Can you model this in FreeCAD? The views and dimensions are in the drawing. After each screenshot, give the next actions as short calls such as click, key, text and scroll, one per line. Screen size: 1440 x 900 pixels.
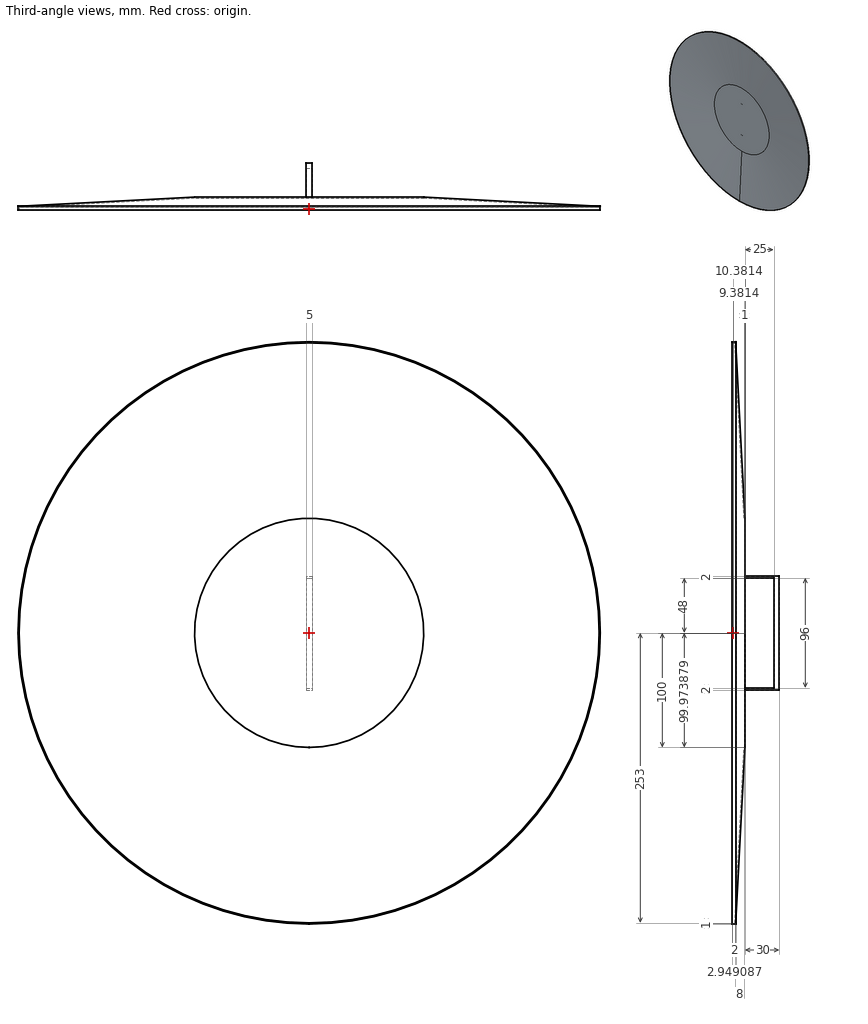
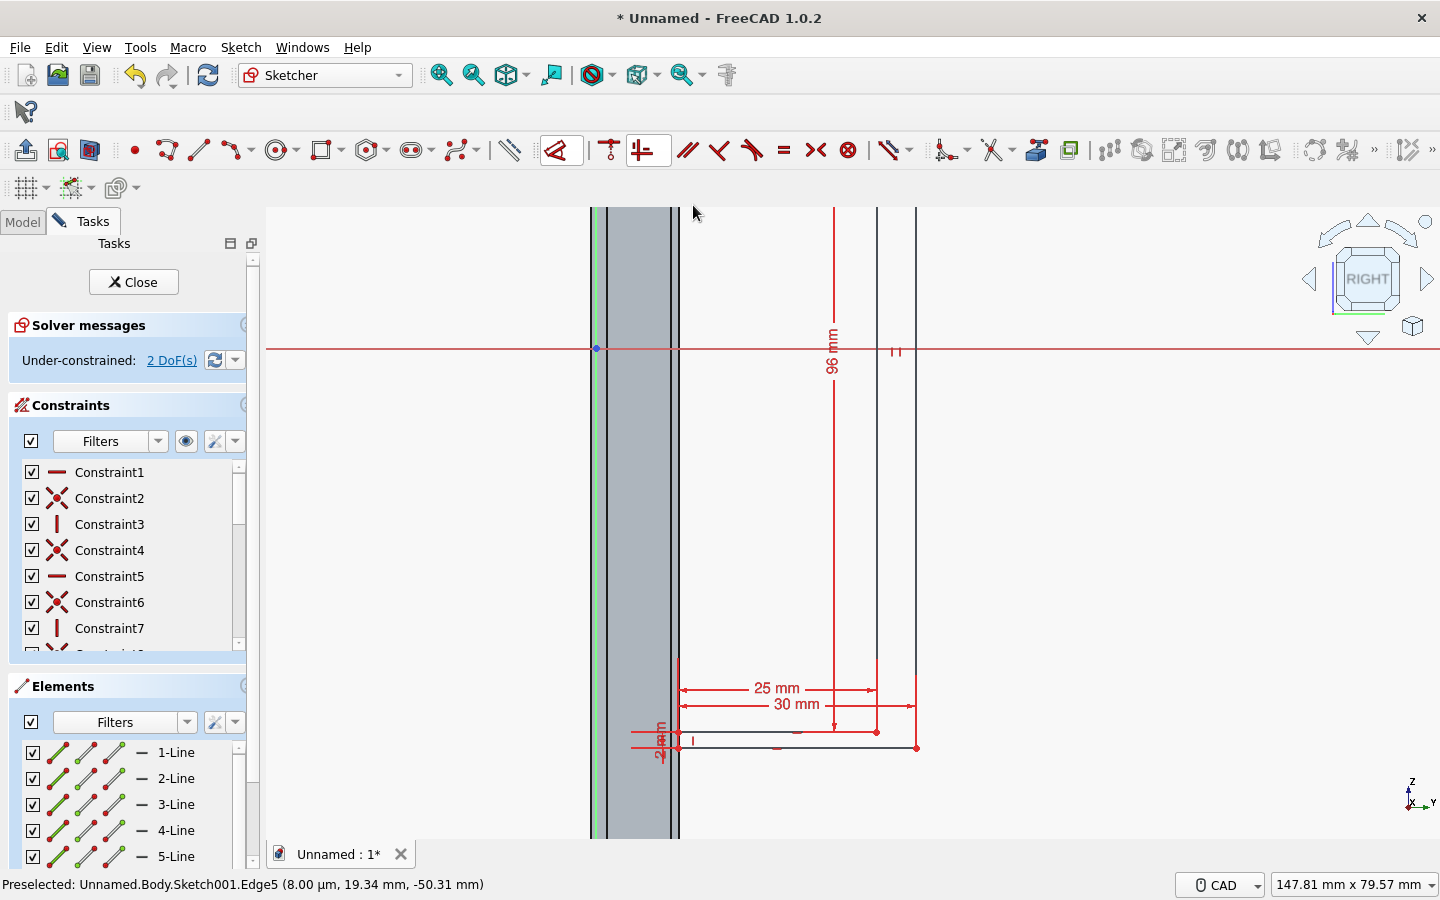
scroll(818, 735, down, 3)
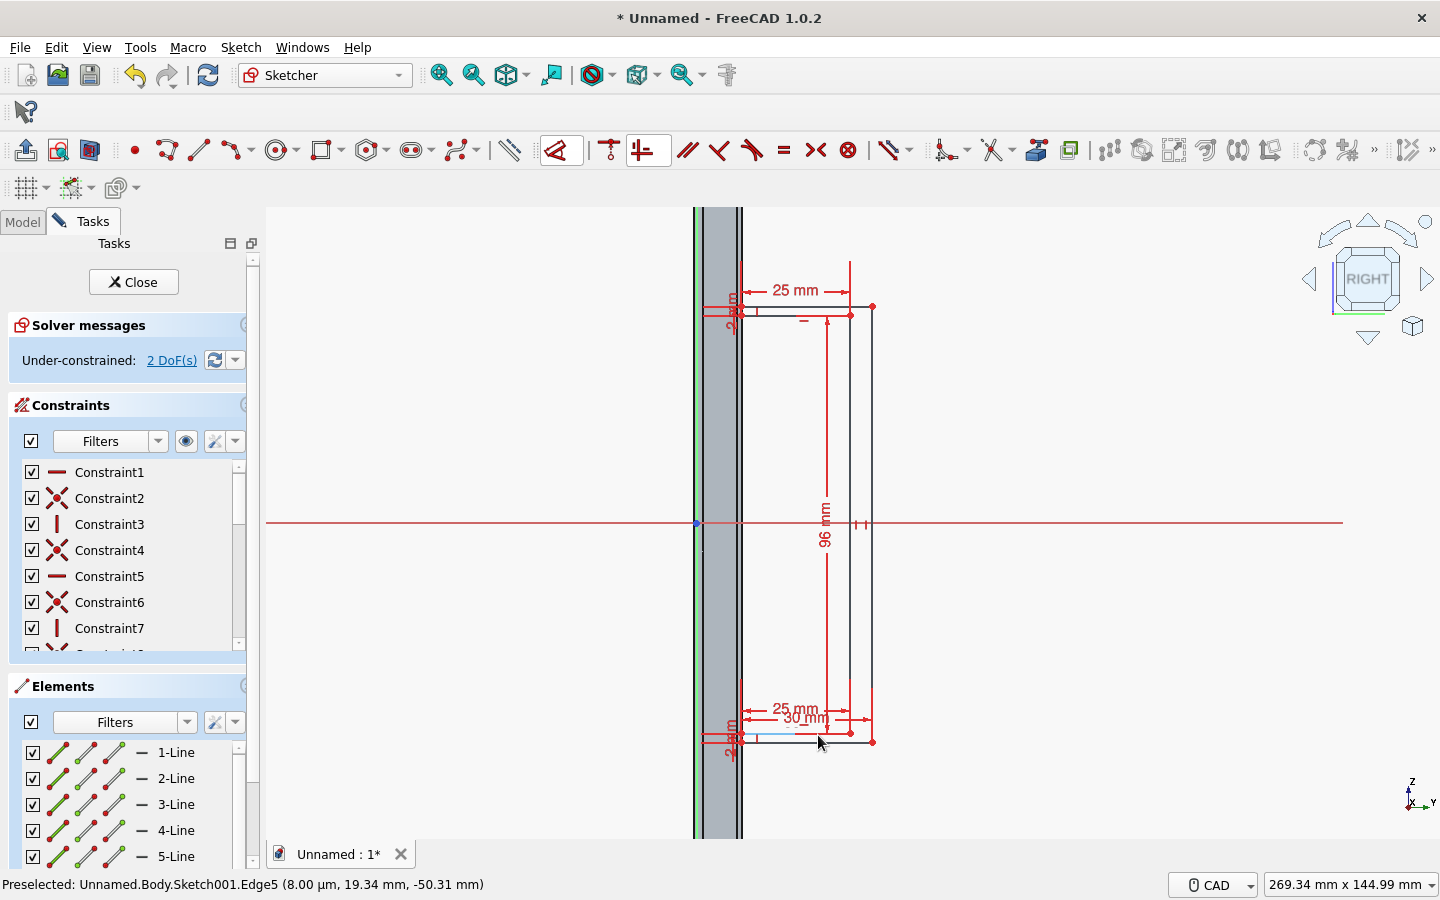
scroll(741, 316, up, 2)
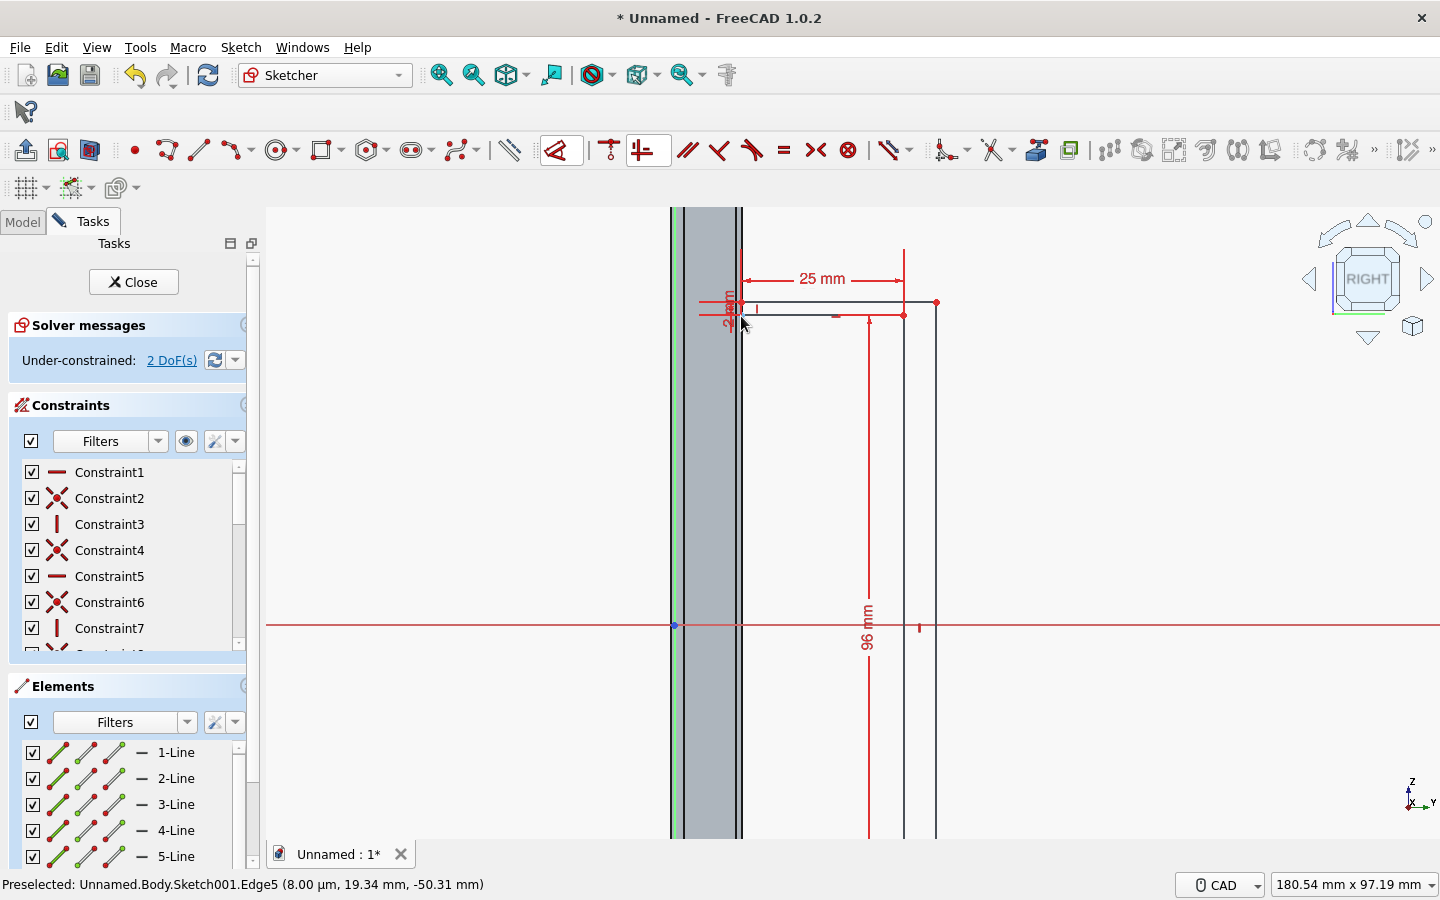
click(741, 315)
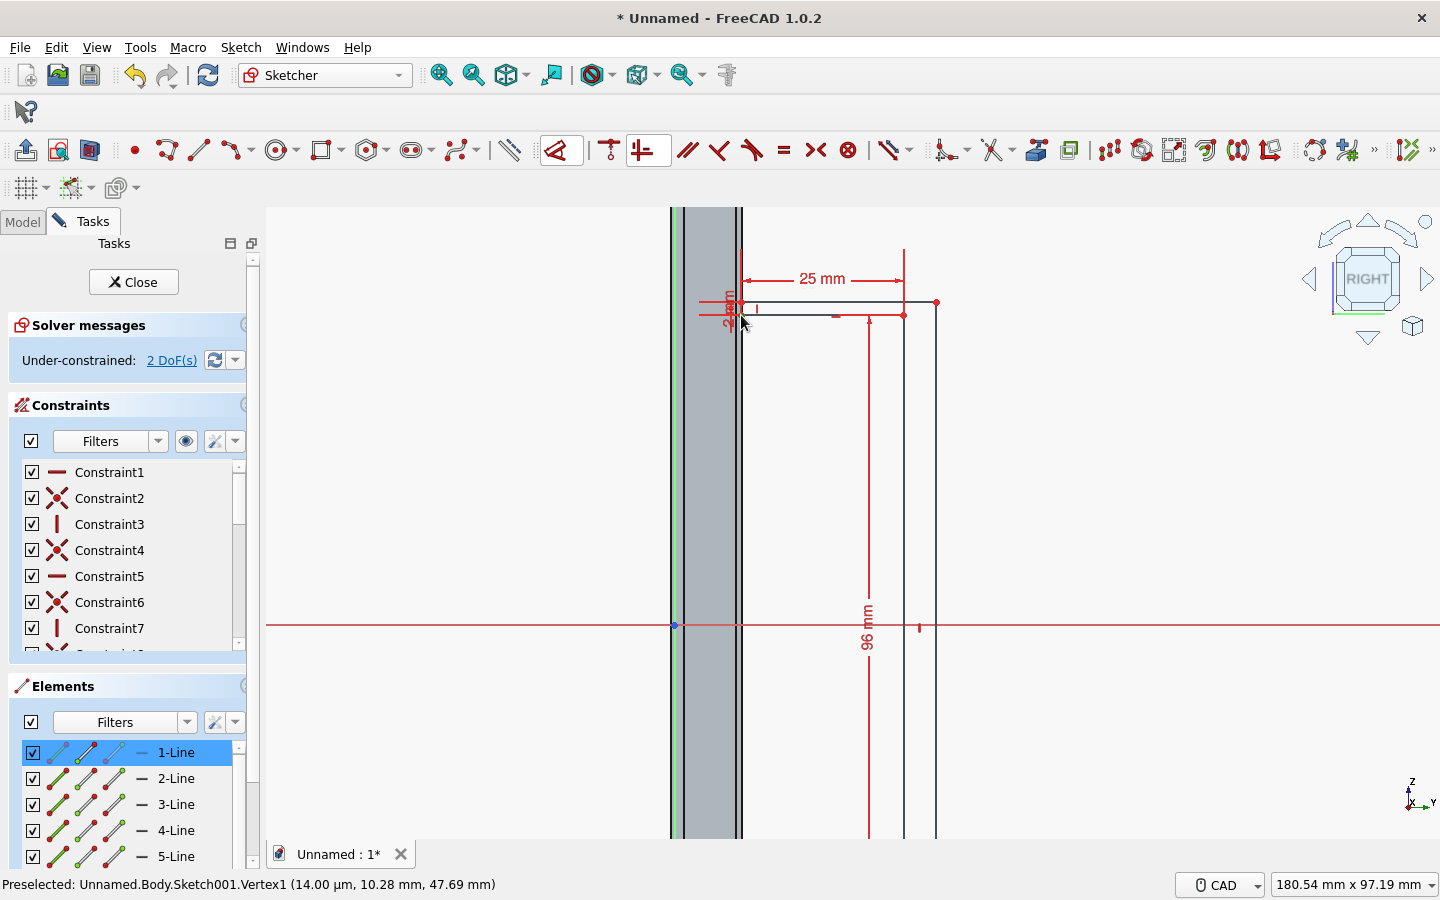
key(i)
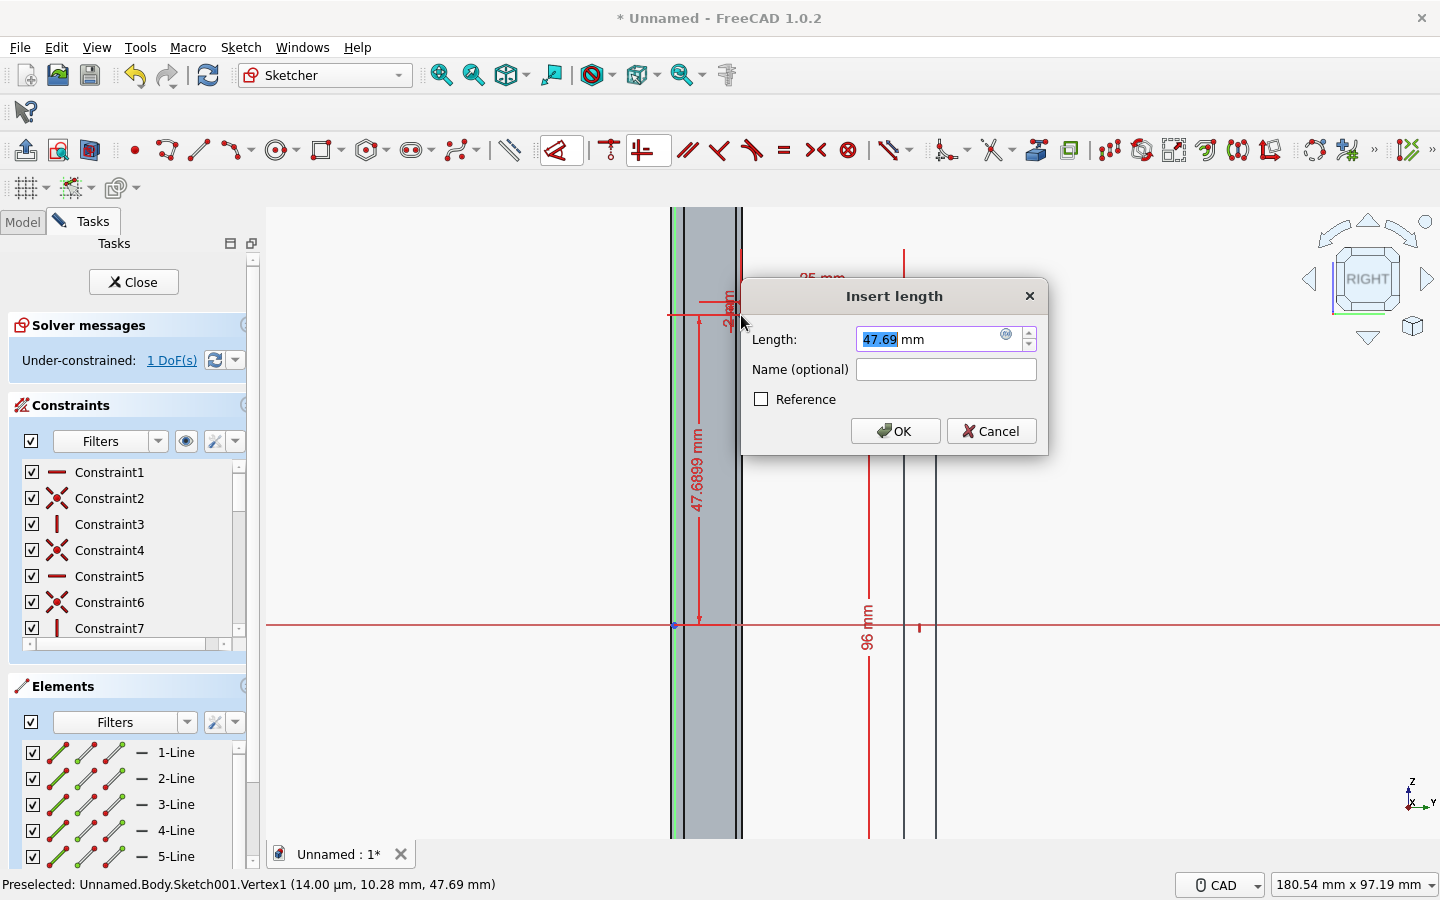
text(48)
key(Return)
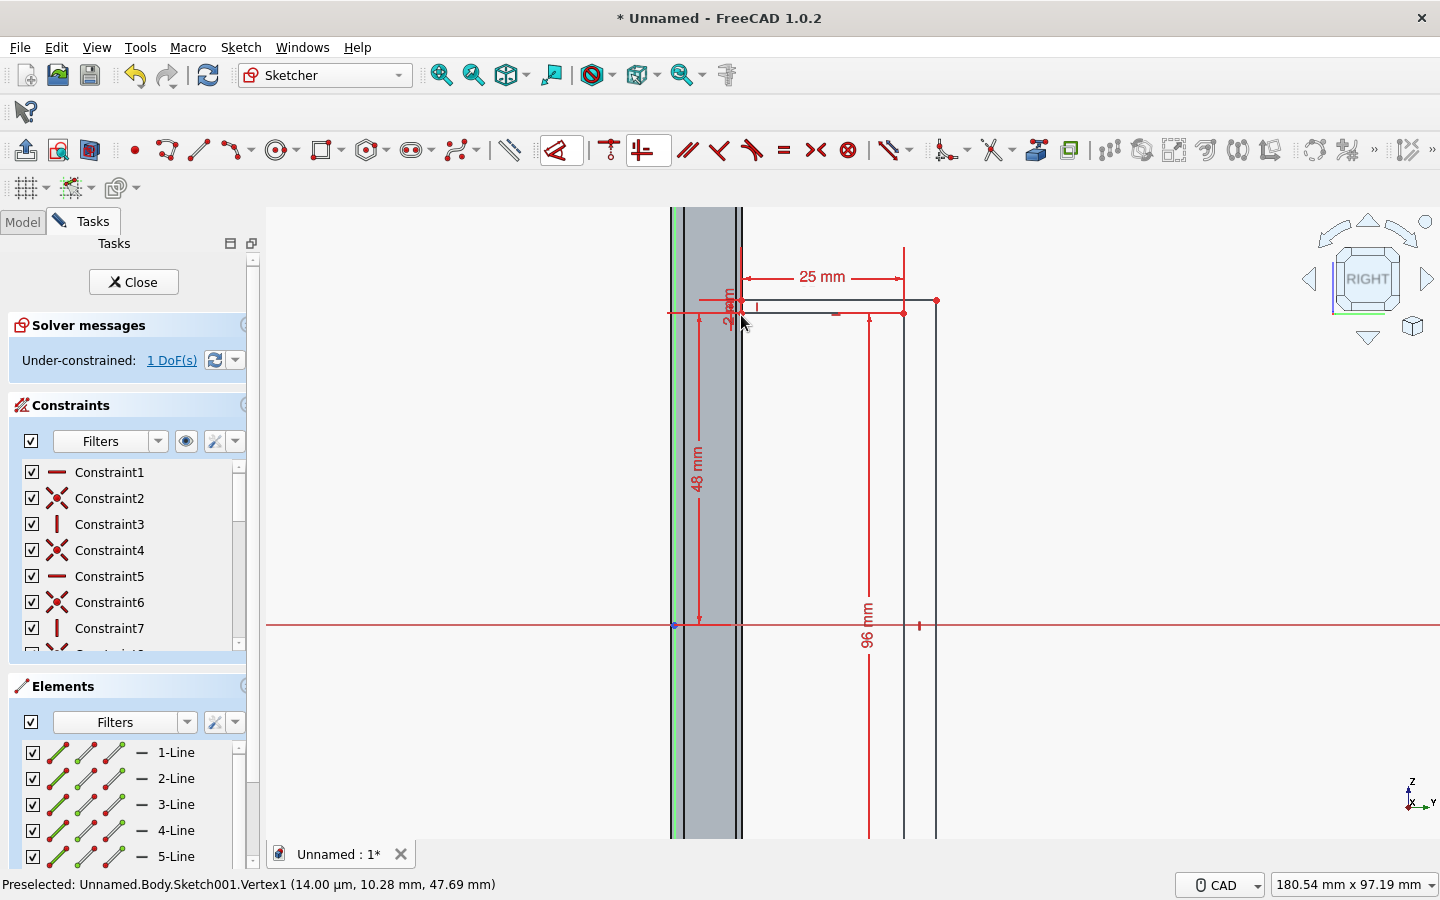
click(741, 313)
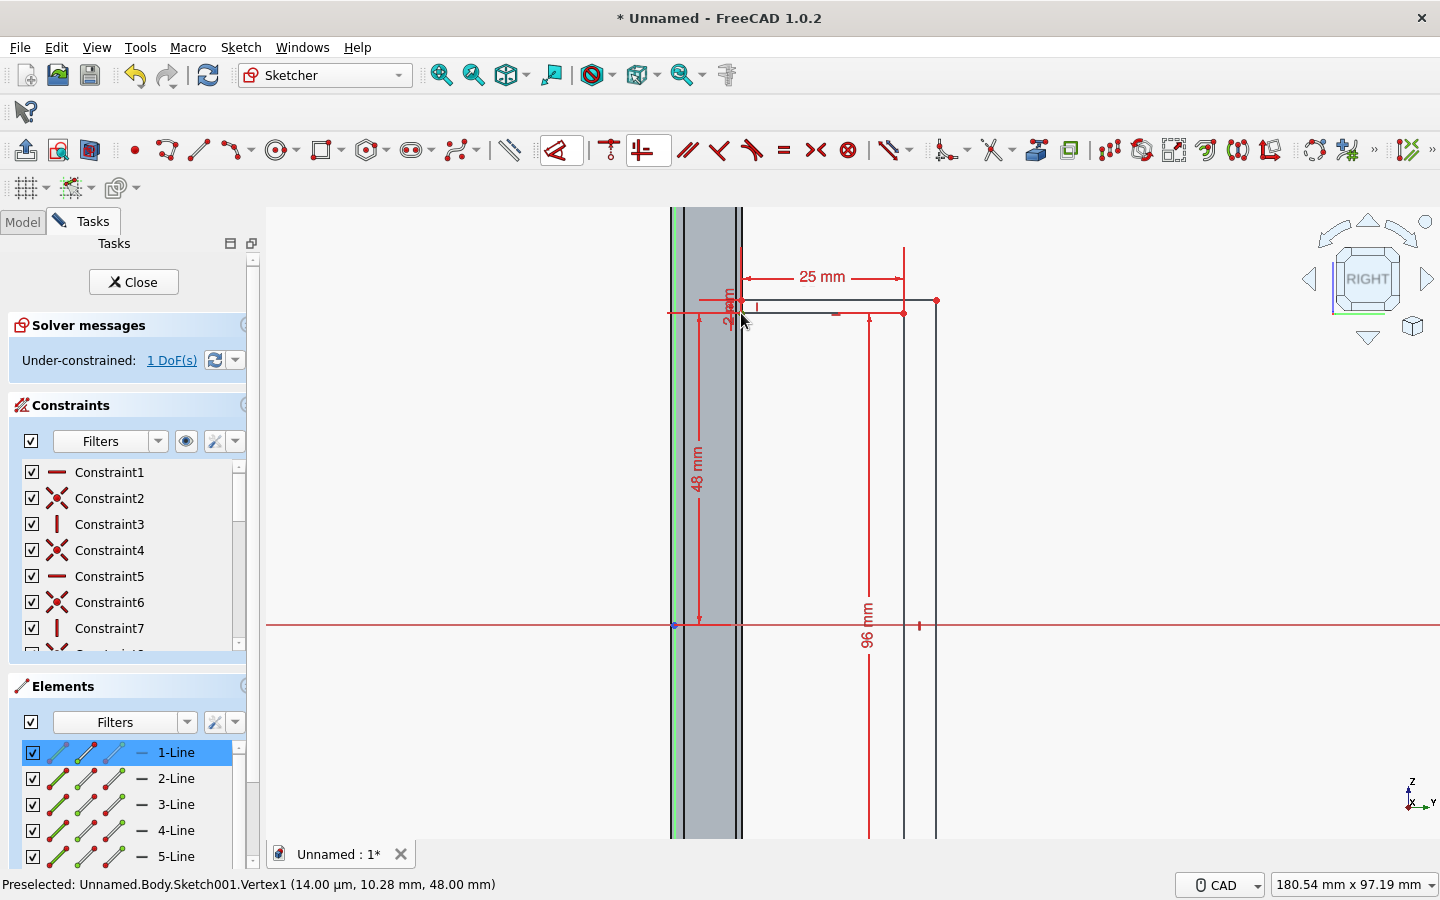
click(578, 150)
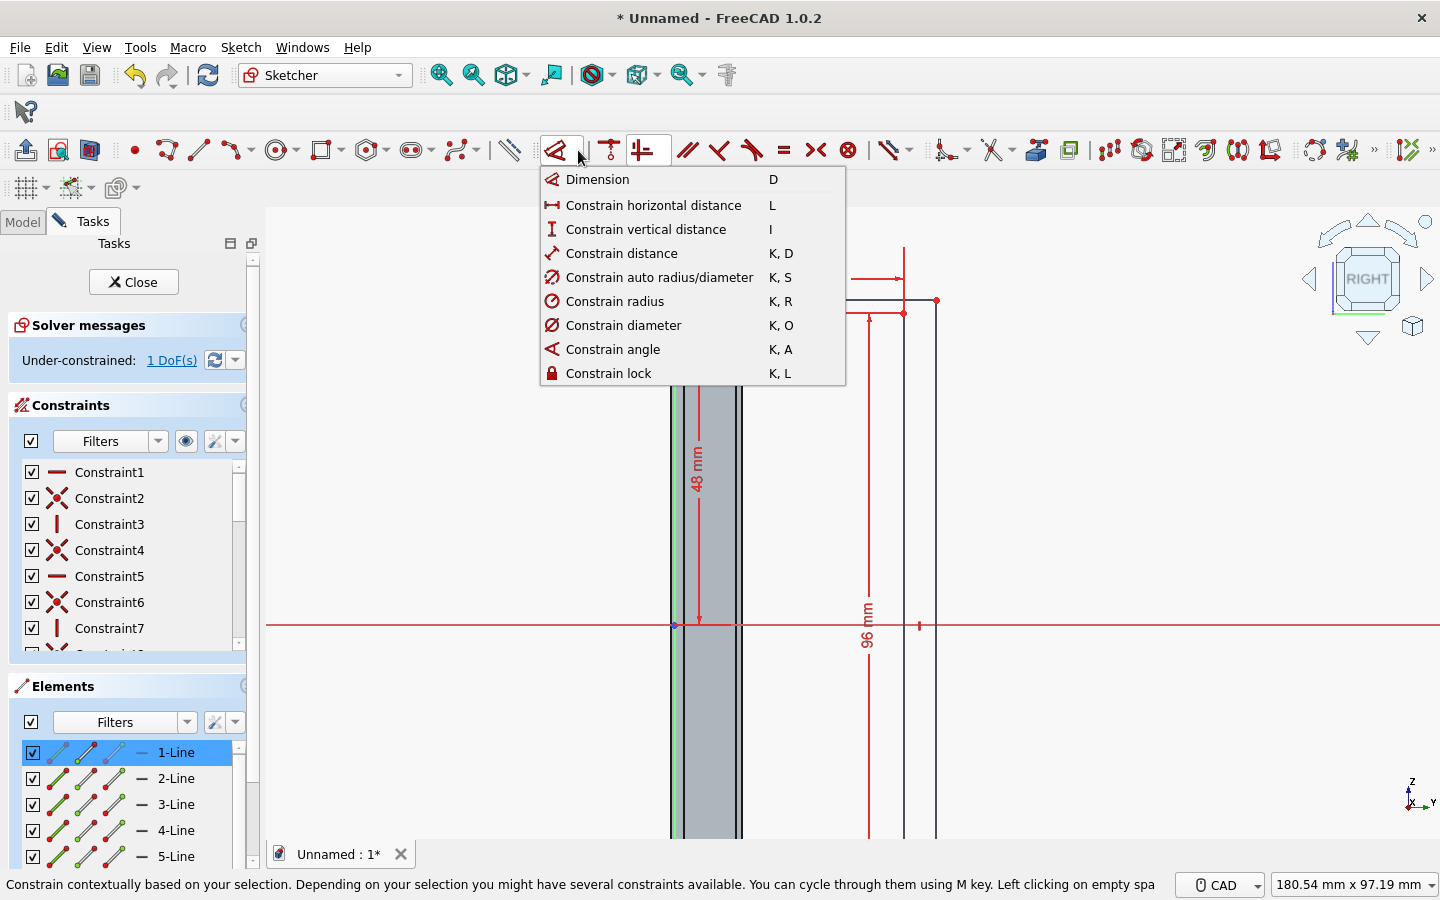
click(693, 205)